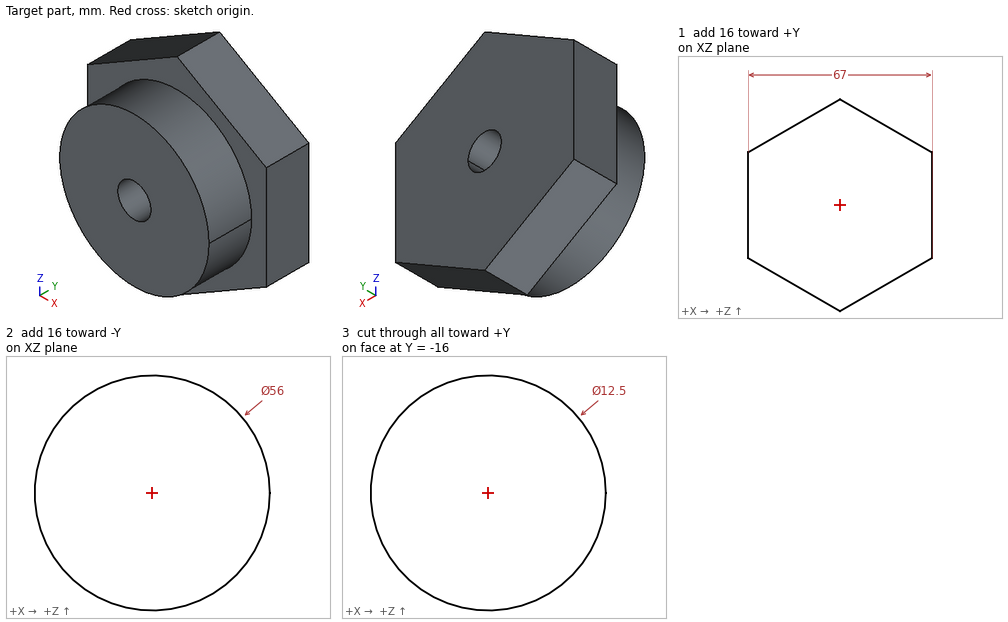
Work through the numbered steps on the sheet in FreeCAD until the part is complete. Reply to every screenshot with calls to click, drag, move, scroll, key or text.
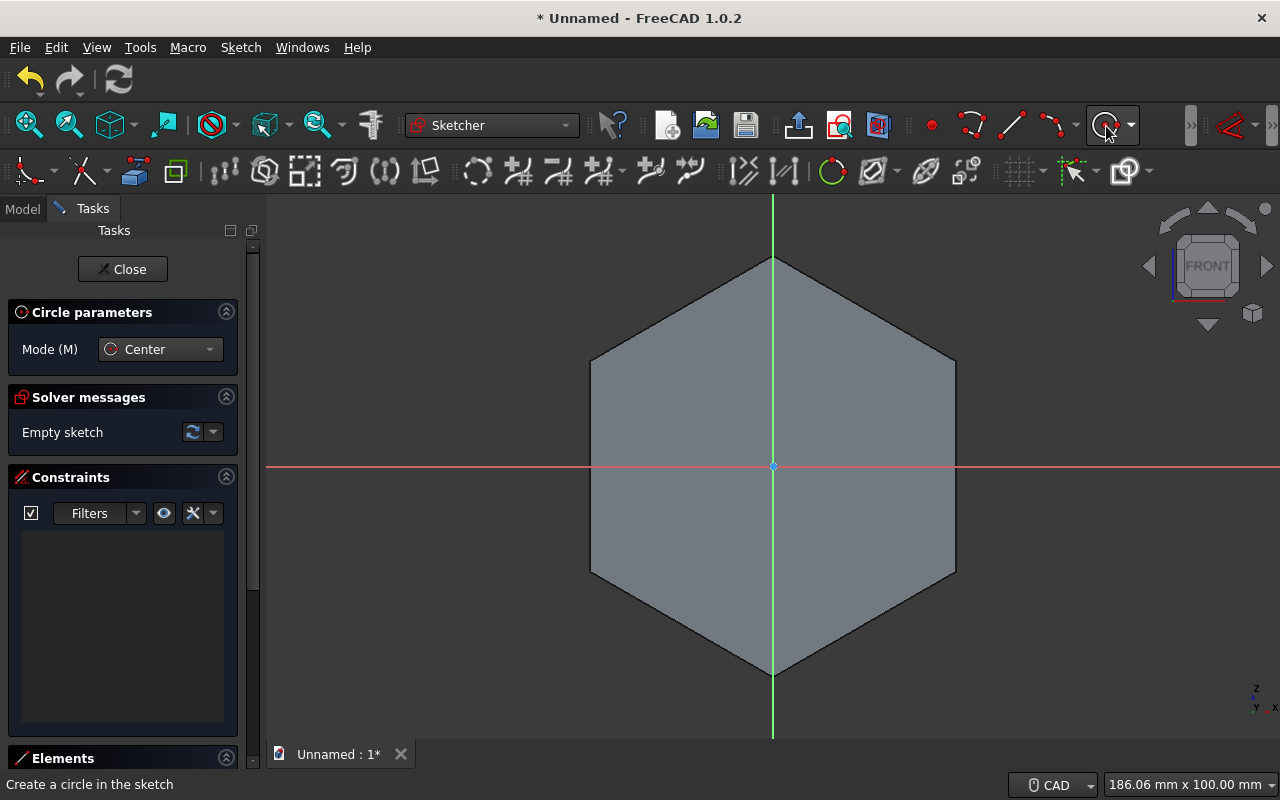
click(773, 466)
click(881, 359)
key(Escape)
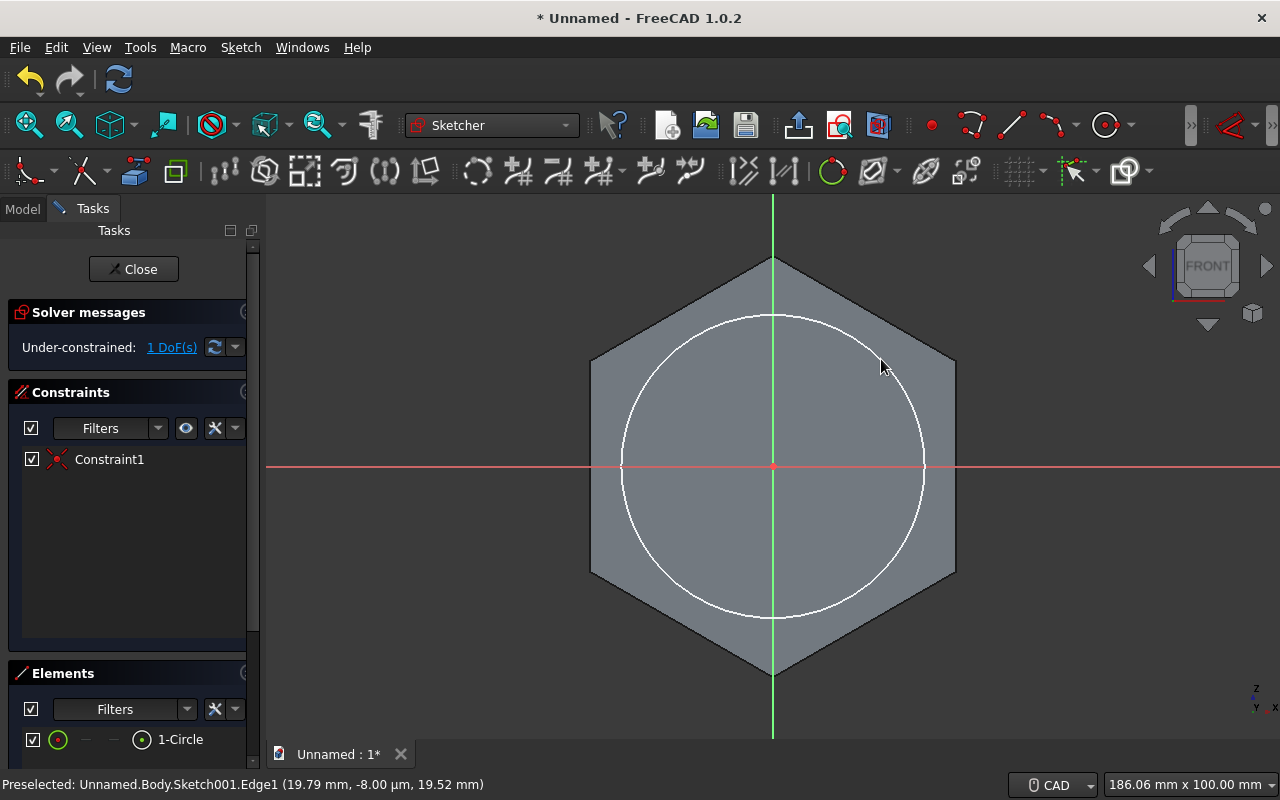
click(1230, 126)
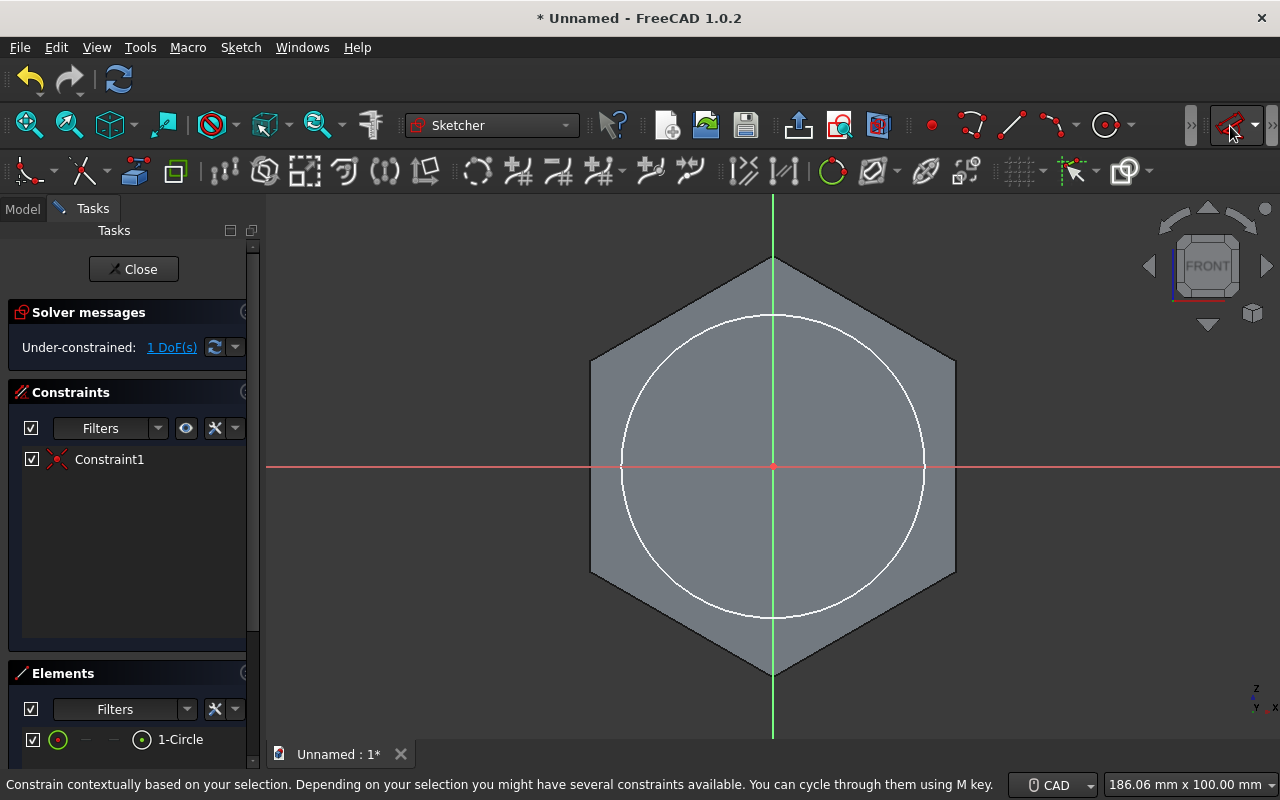
click(880, 359)
click(903, 336)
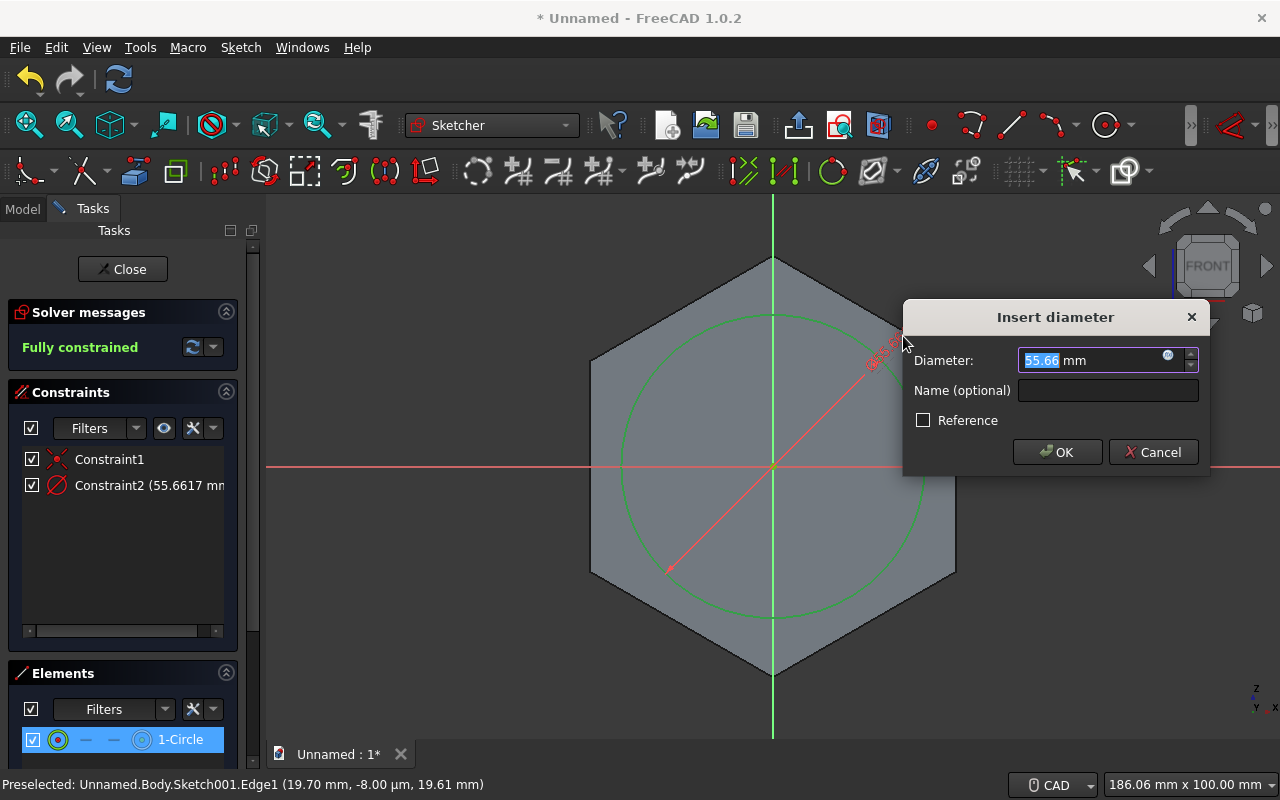
text(56)
key(Return)
key(Escape)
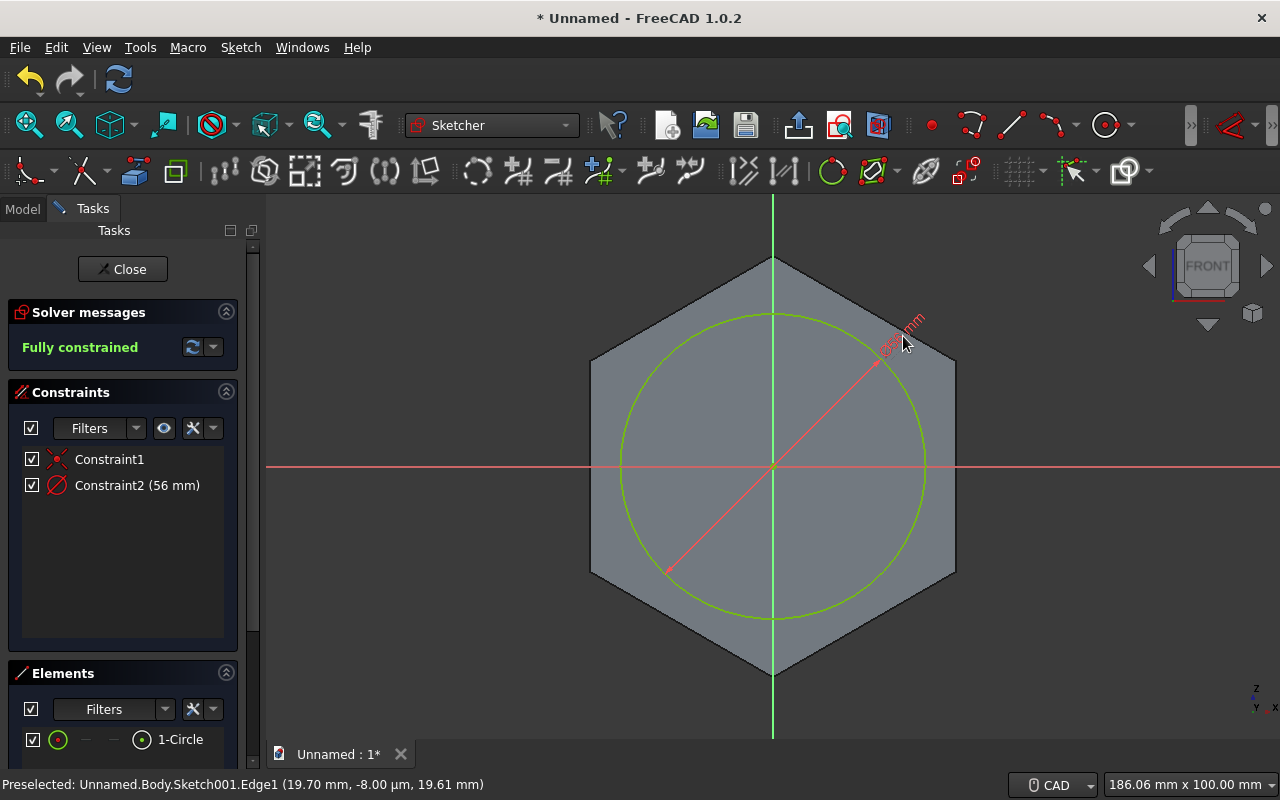
click(123, 269)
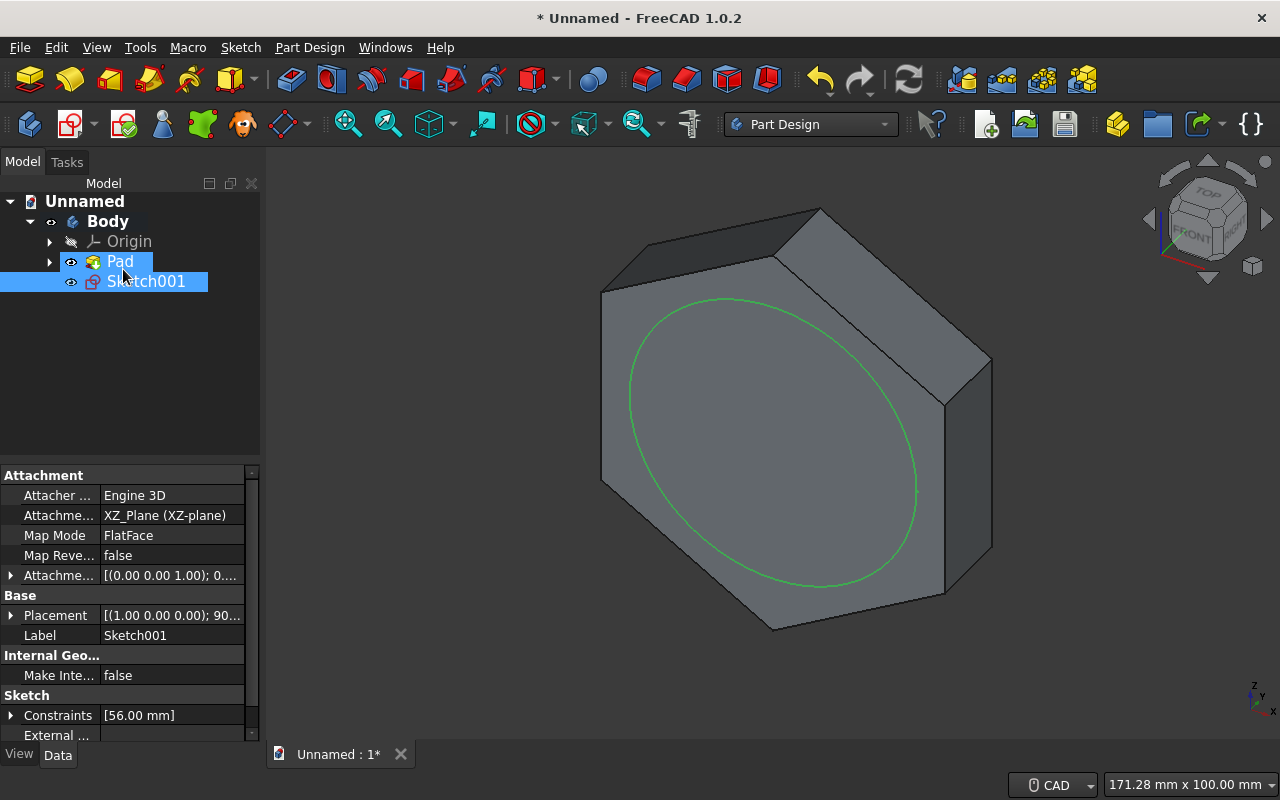
click(30, 80)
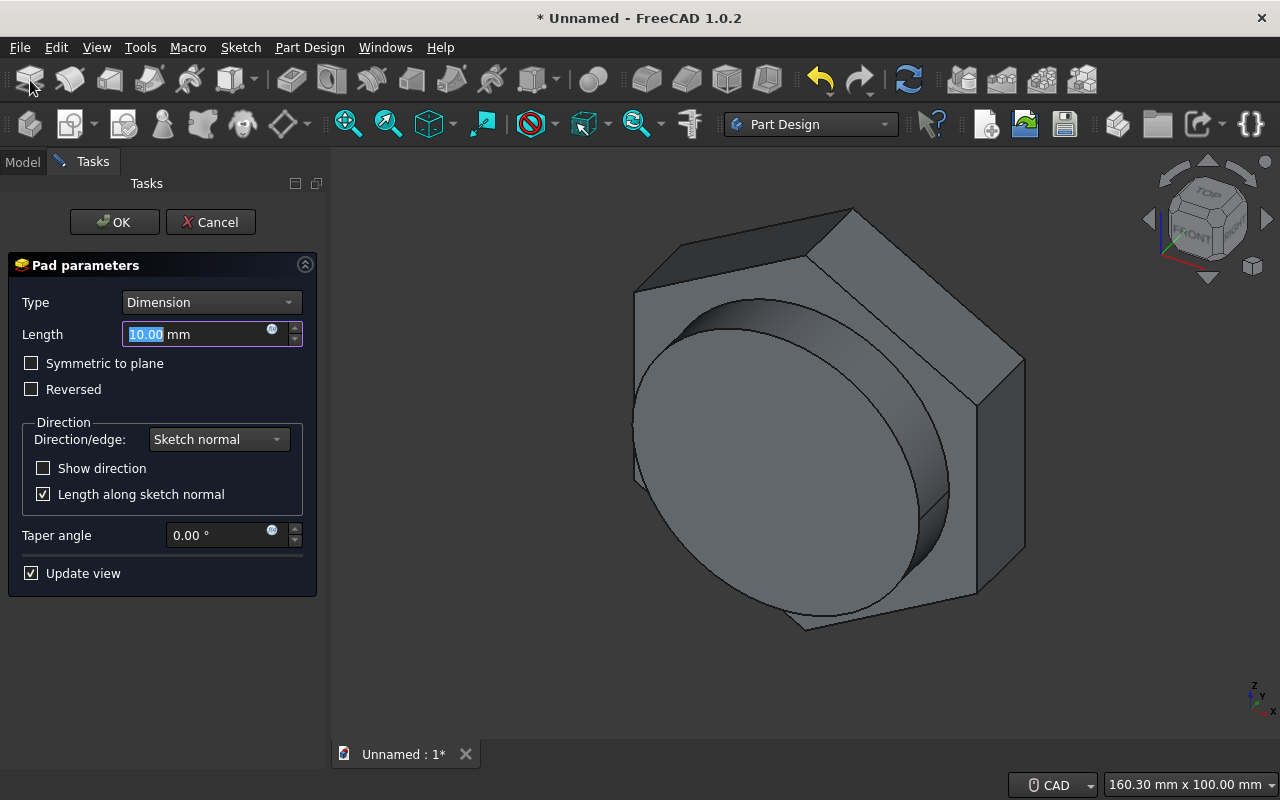
text(16)
key(Tab)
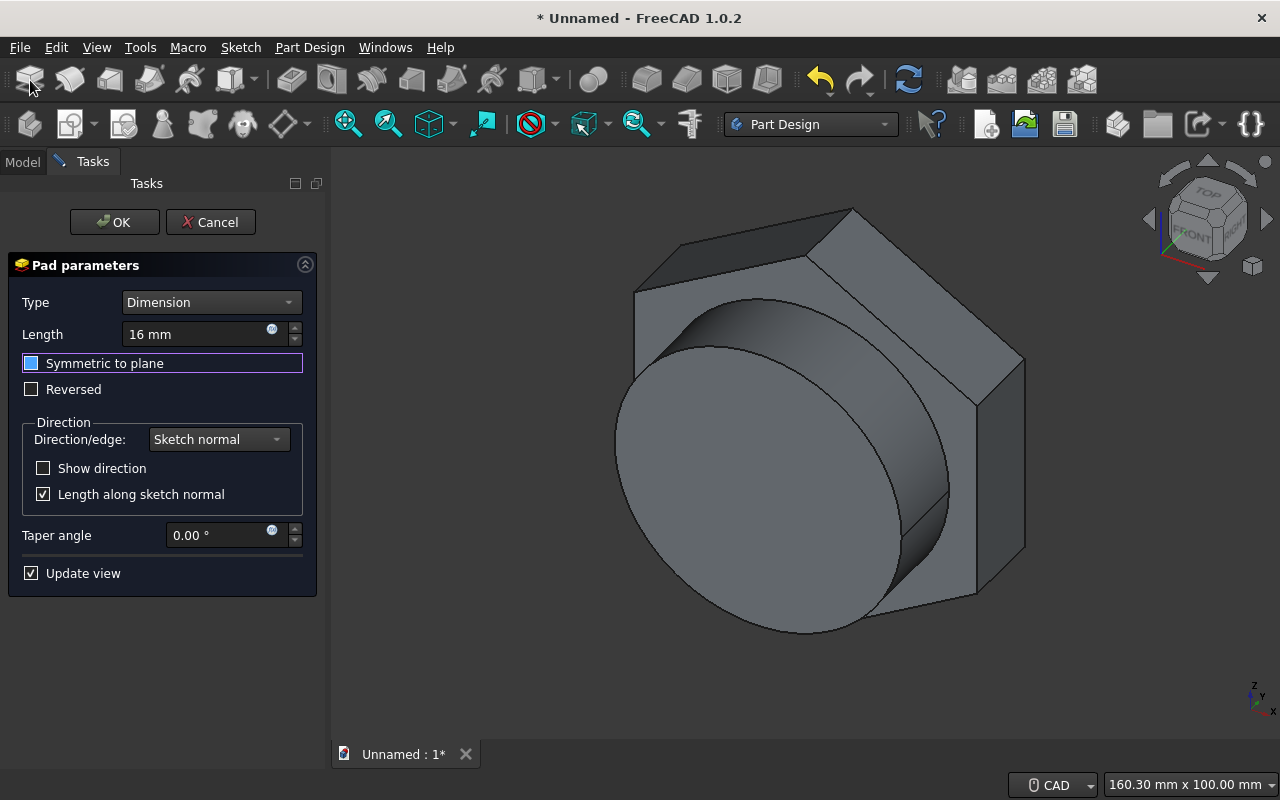
click(115, 222)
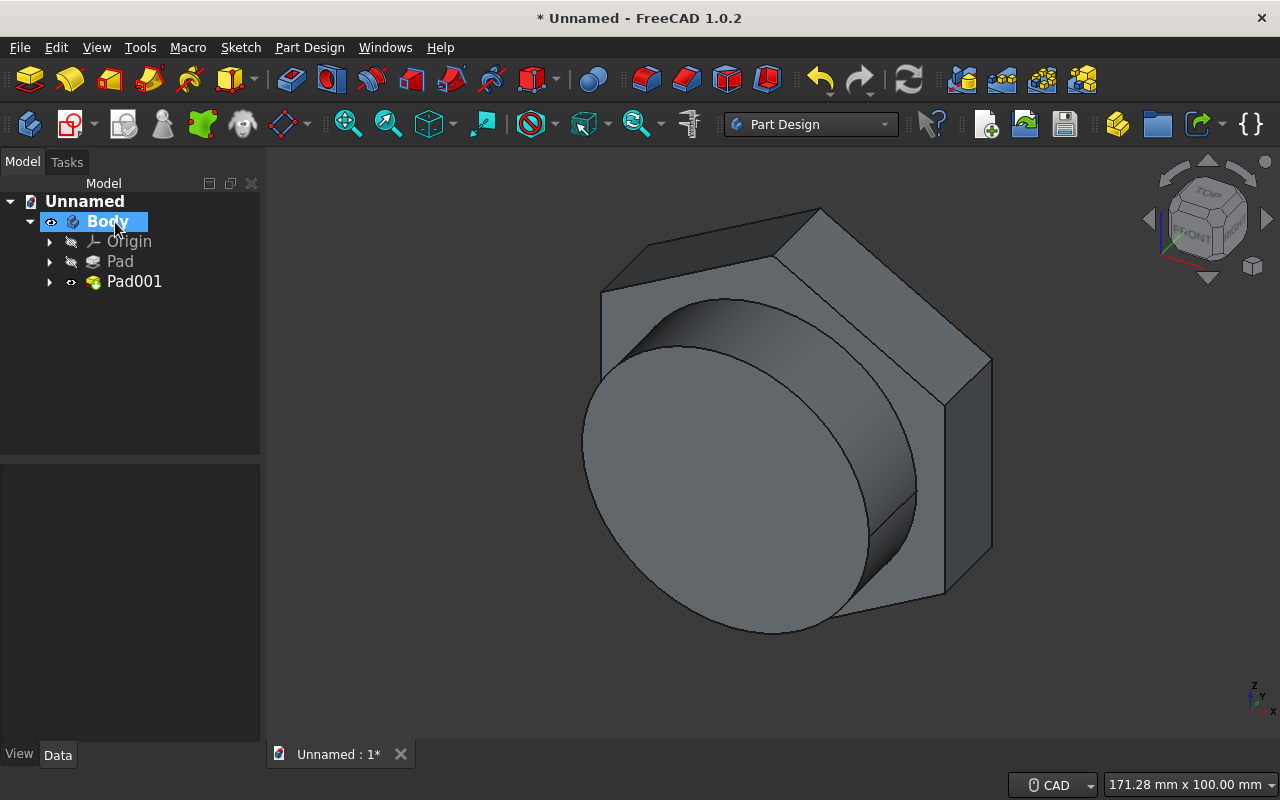
click(726, 489)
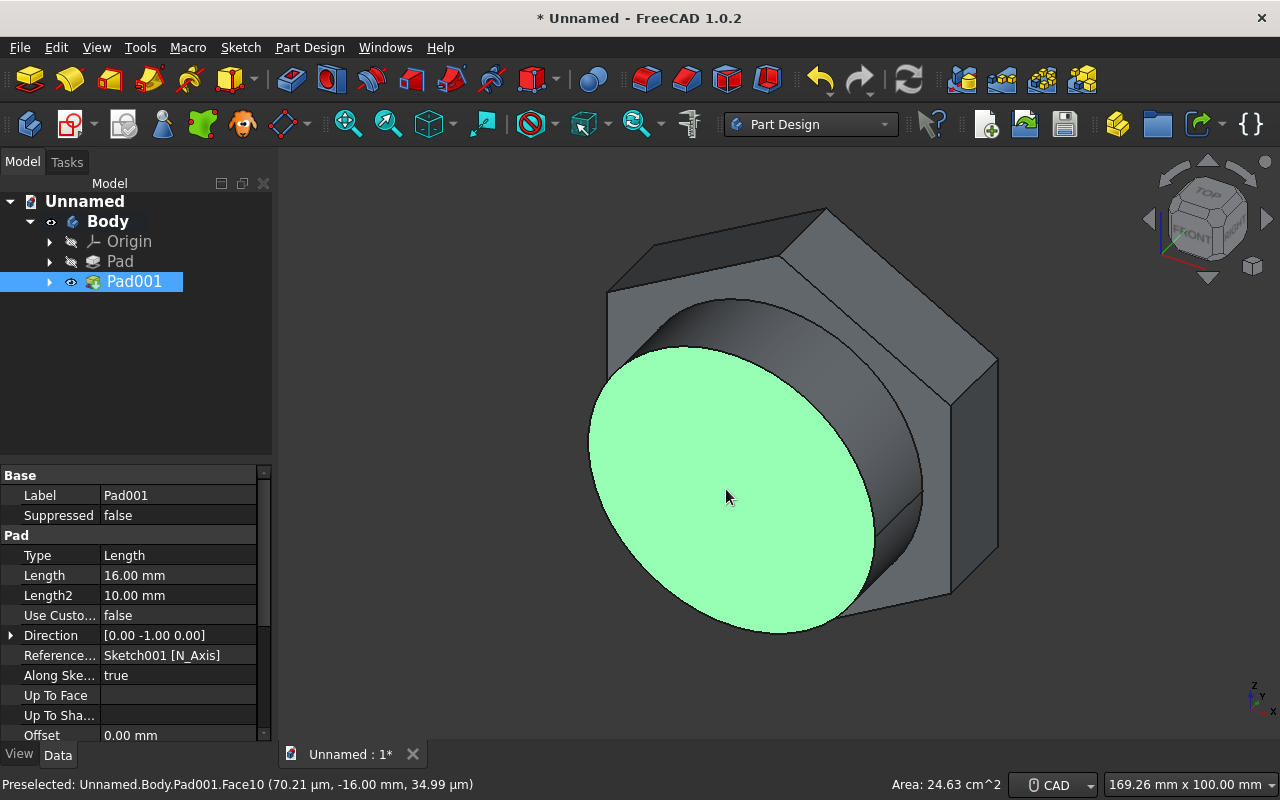
click(70, 124)